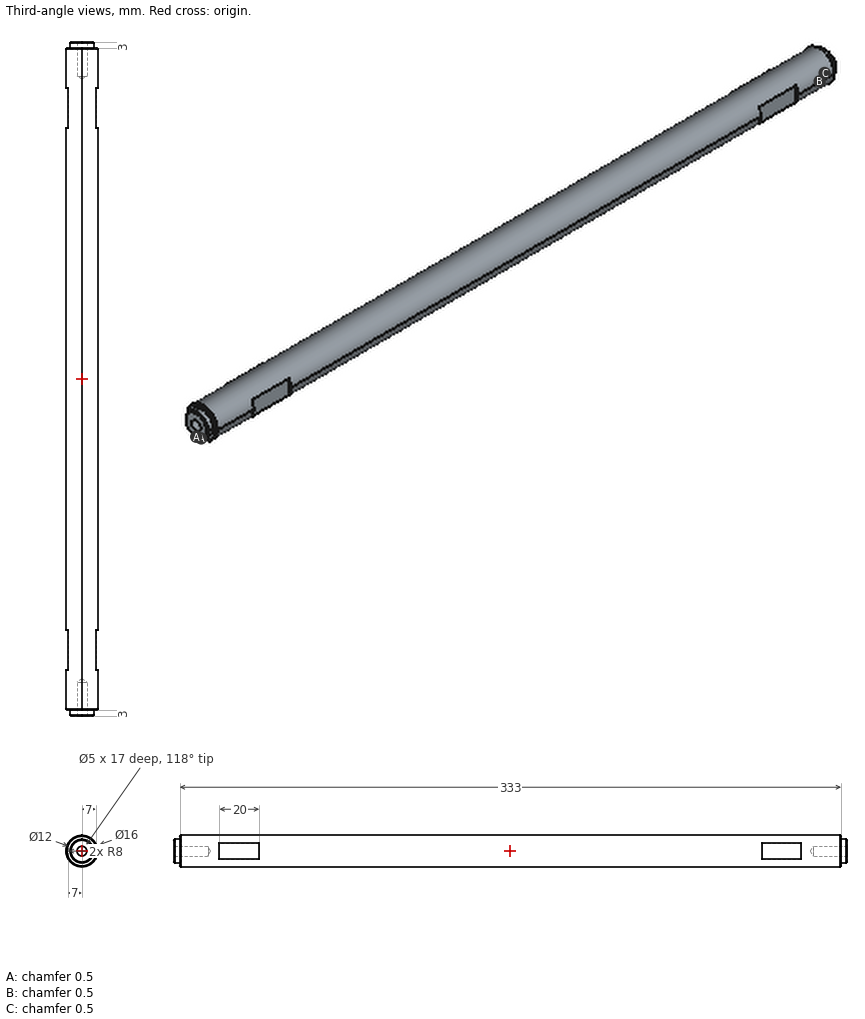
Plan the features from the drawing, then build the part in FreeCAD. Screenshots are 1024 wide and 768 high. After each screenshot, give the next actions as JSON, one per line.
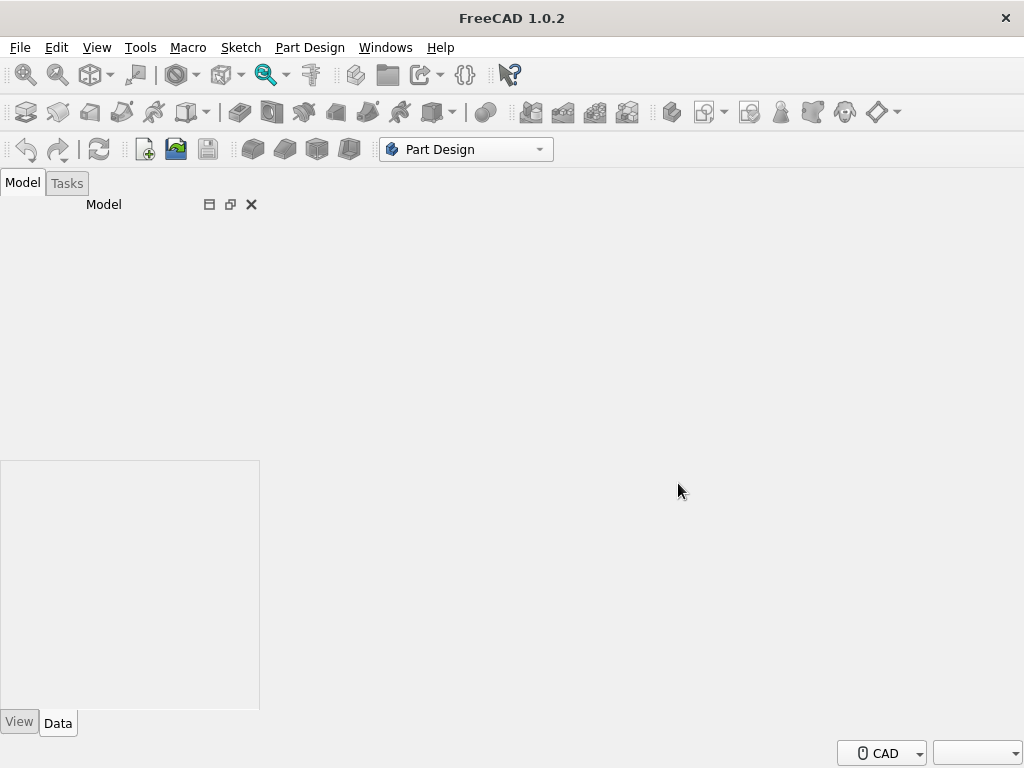
{"action": "left_click", "coordinate": [144, 150]}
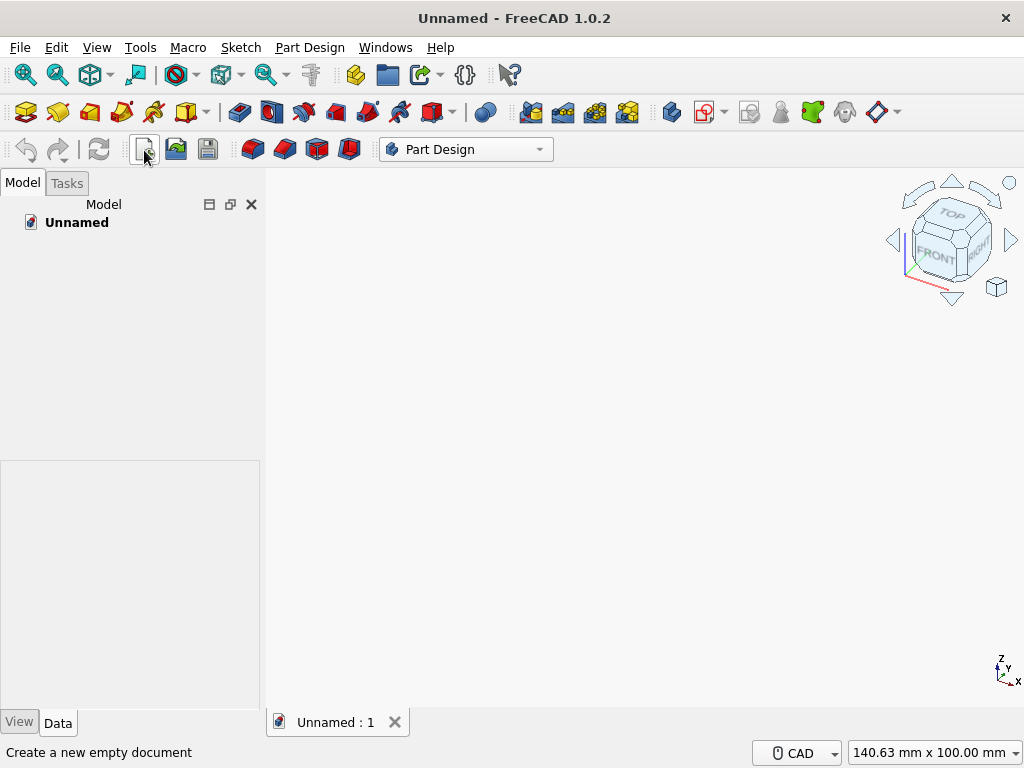
{"action": "left_click", "coordinate": [704, 112]}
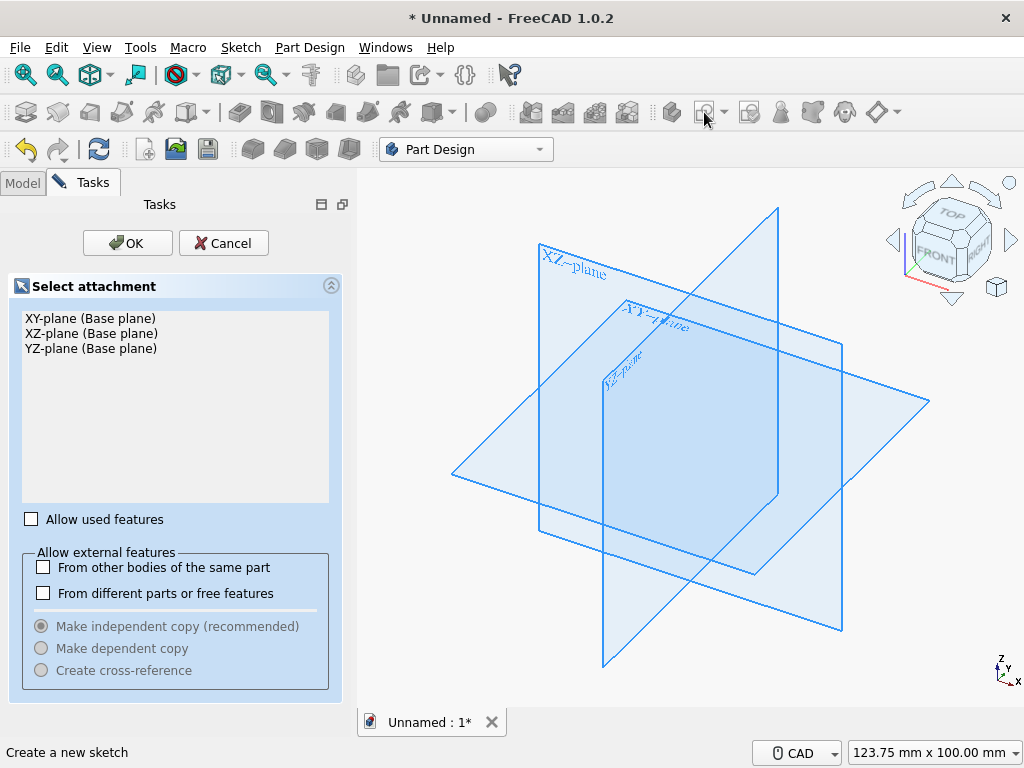
{"action": "left_click", "coordinate": [82, 334]}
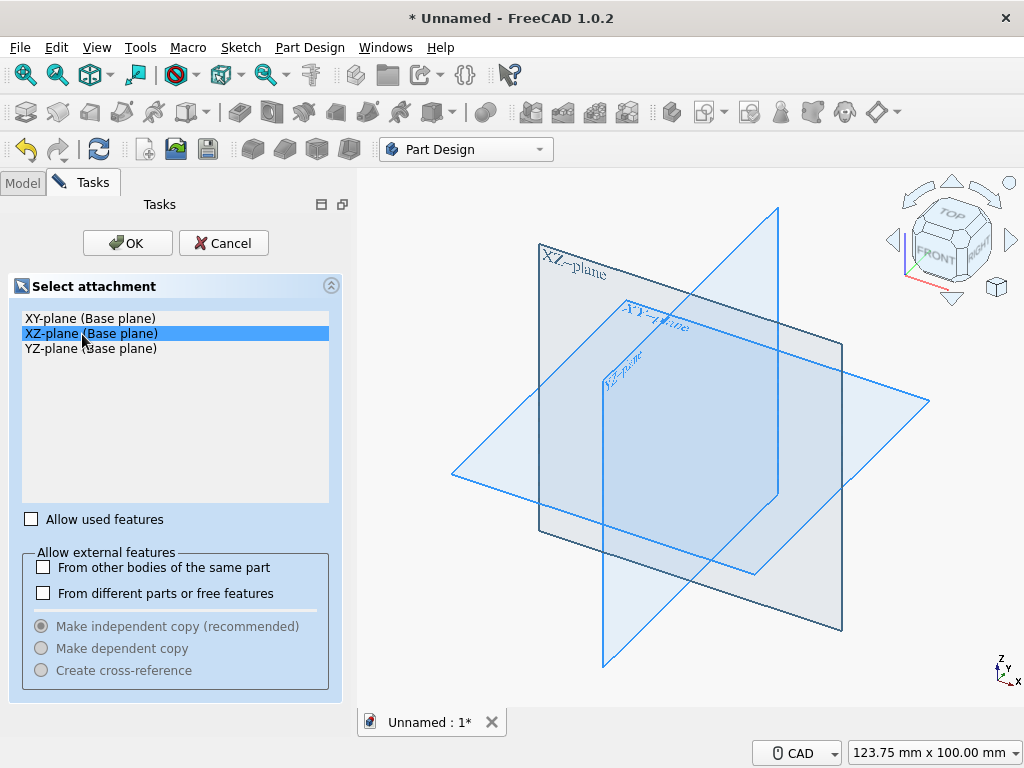
{"action": "left_click", "coordinate": [128, 243]}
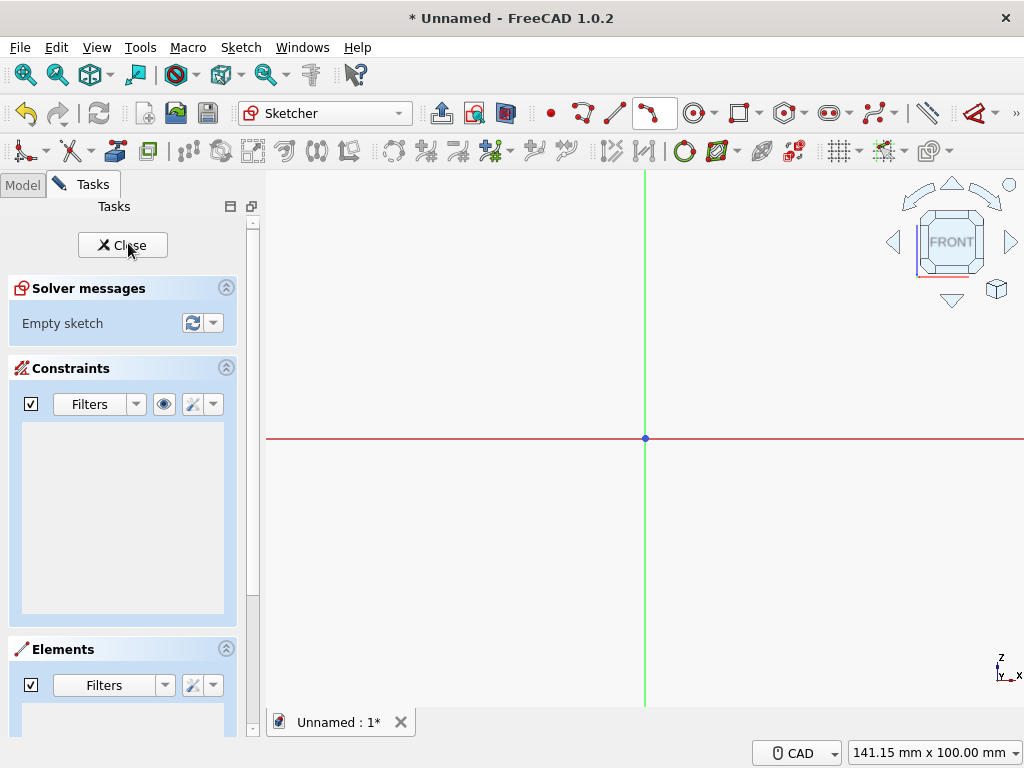
{"action": "scroll", "coordinate": [667, 438], "scroll_direction": "up", "scroll_amount": 7}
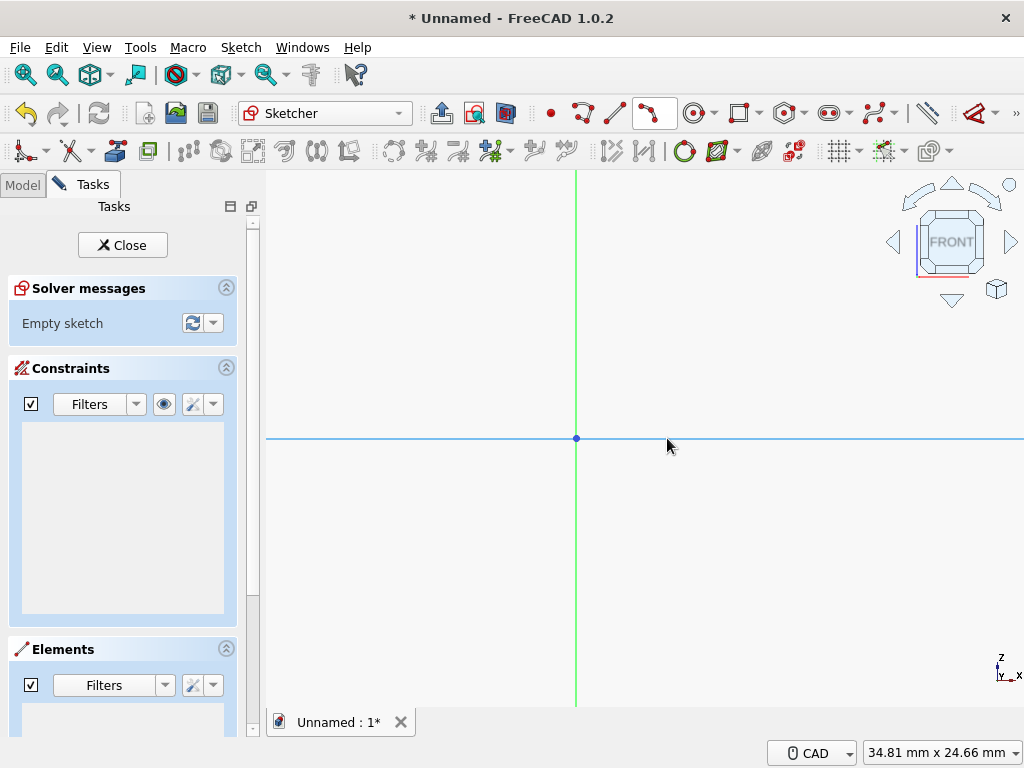
{"action": "key", "text": "g c"}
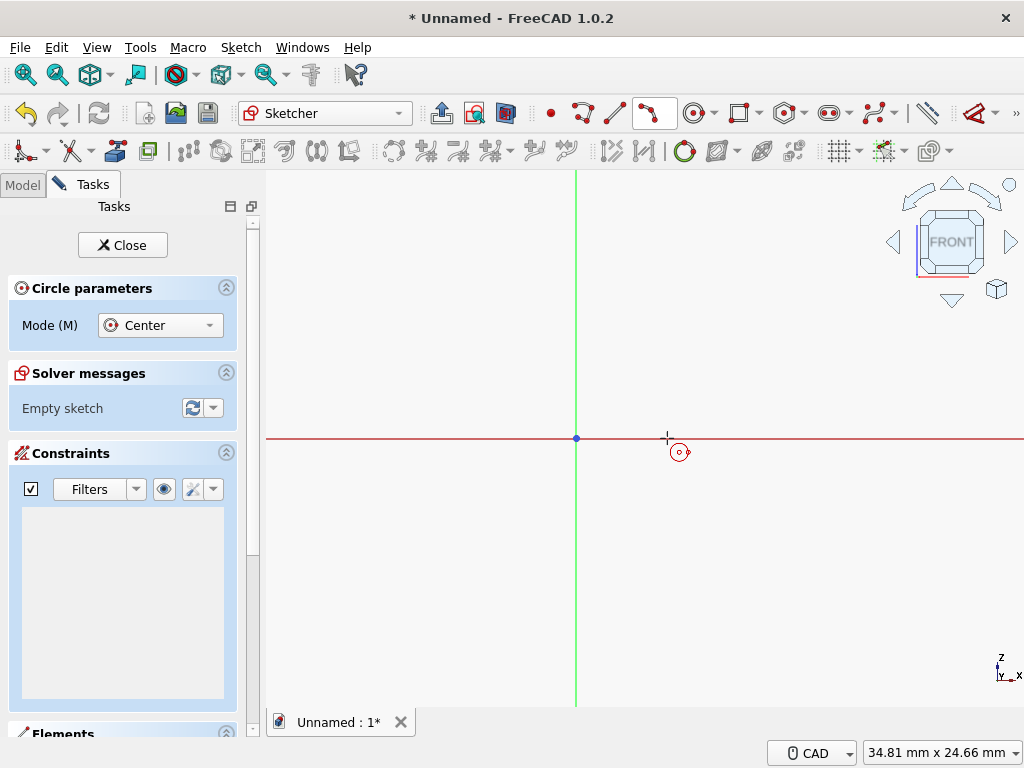
{"action": "left_click", "coordinate": [576, 438]}
{"action": "left_click", "coordinate": [699, 315]}
{"action": "key", "text": "Escape"}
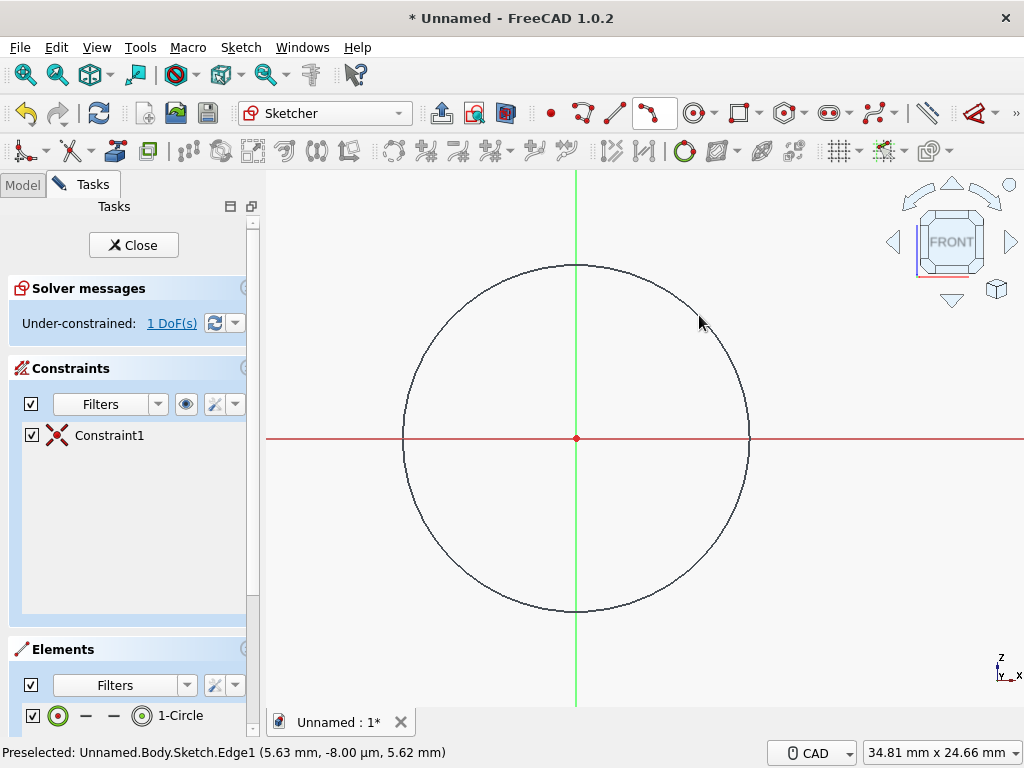
{"action": "left_click", "coordinate": [974, 114]}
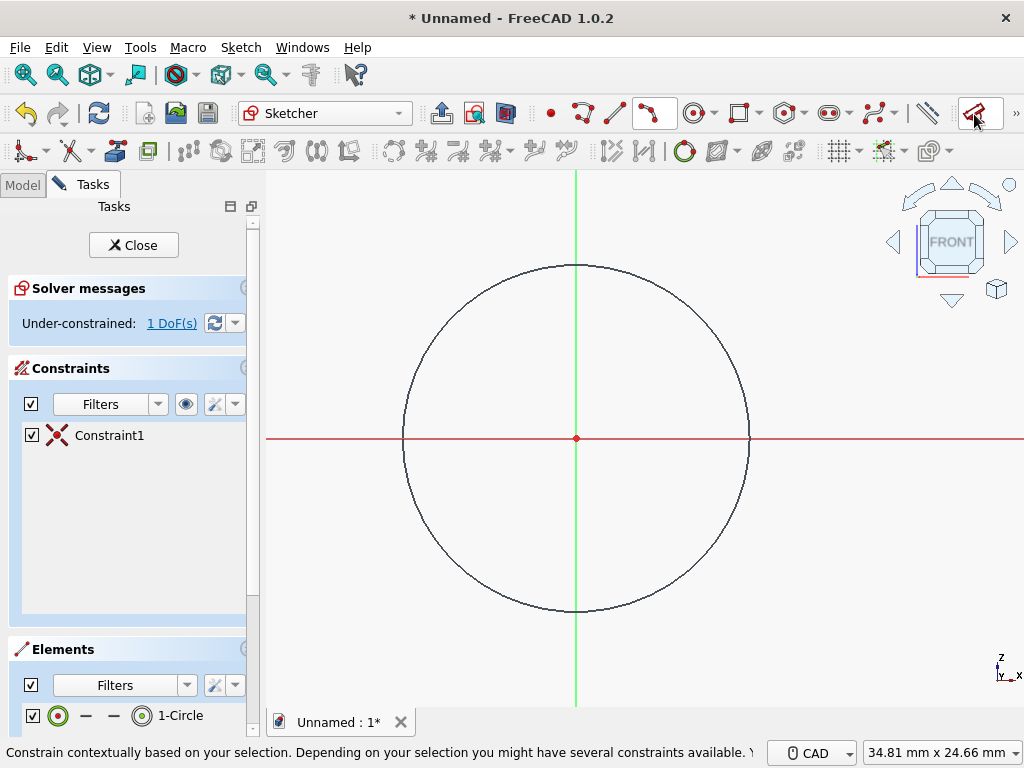
{"action": "left_click", "coordinate": [698, 315]}
{"action": "left_click", "coordinate": [720, 292]}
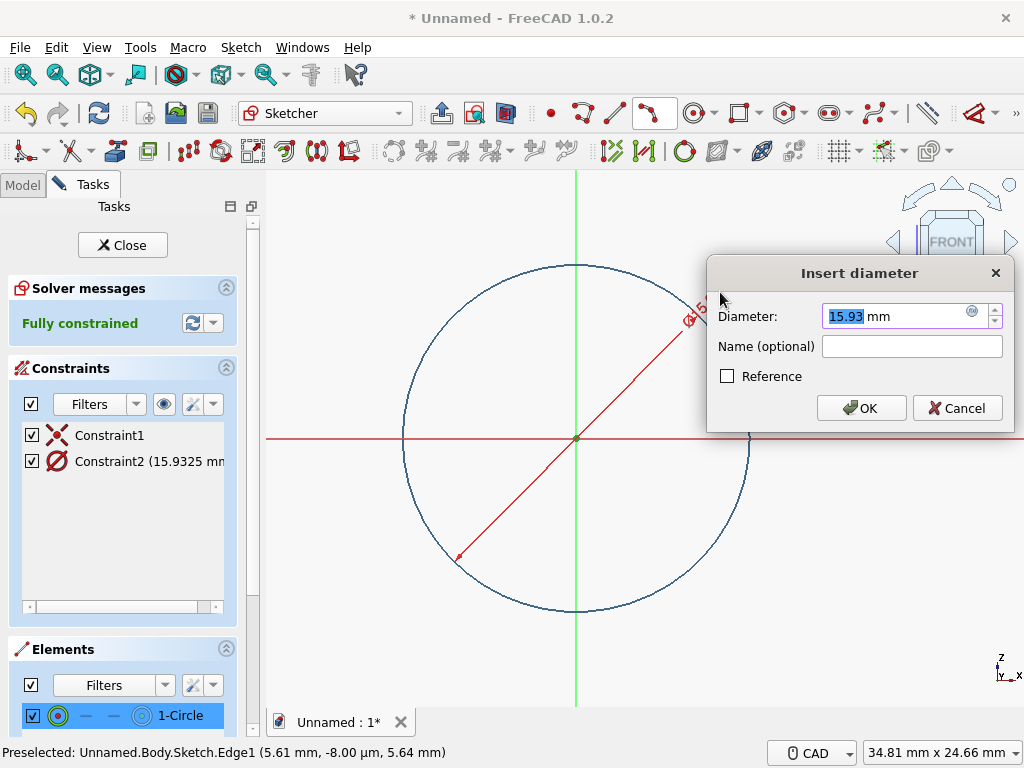
{"action": "type", "text": "16"}
{"action": "key", "text": "Return"}
{"action": "key", "text": "Escape"}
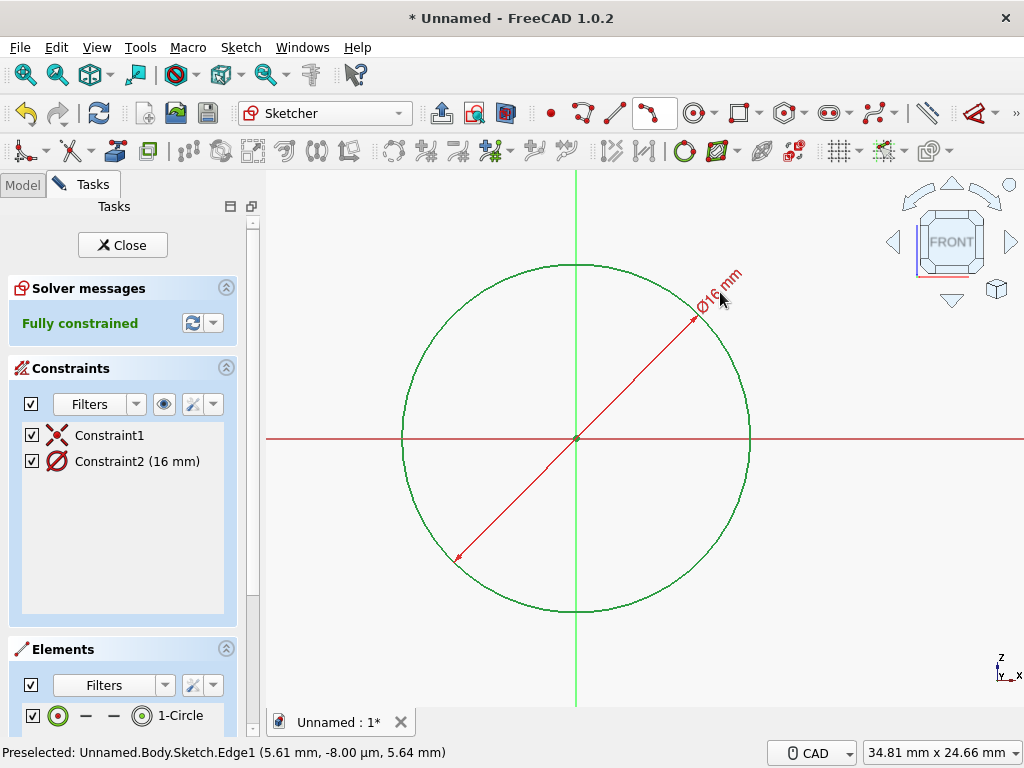
{"action": "left_click", "coordinate": [123, 245]}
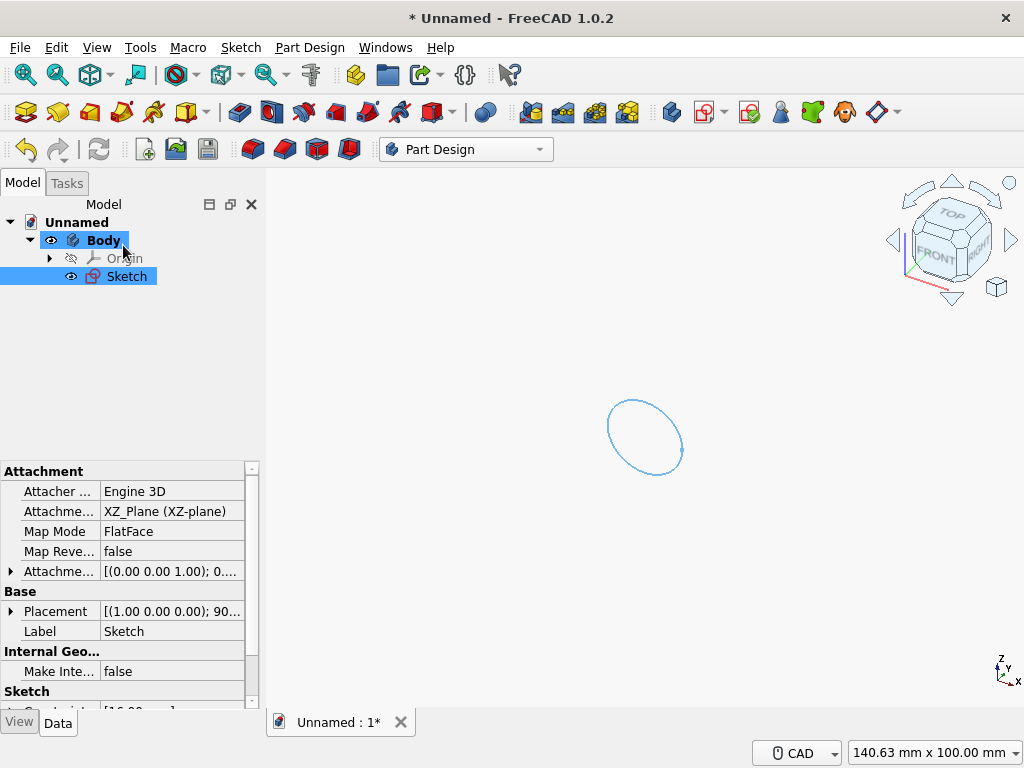
{"action": "left_click", "coordinate": [26, 112]}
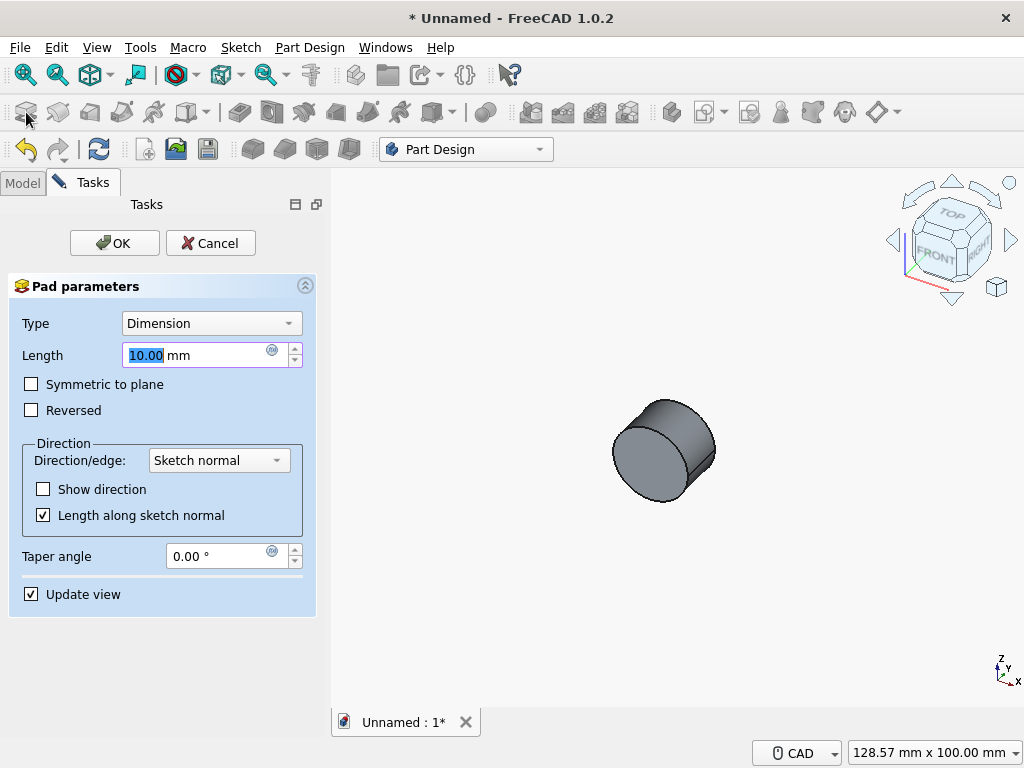
{"action": "type", "text": "333"}
{"action": "key", "text": "Tab"}